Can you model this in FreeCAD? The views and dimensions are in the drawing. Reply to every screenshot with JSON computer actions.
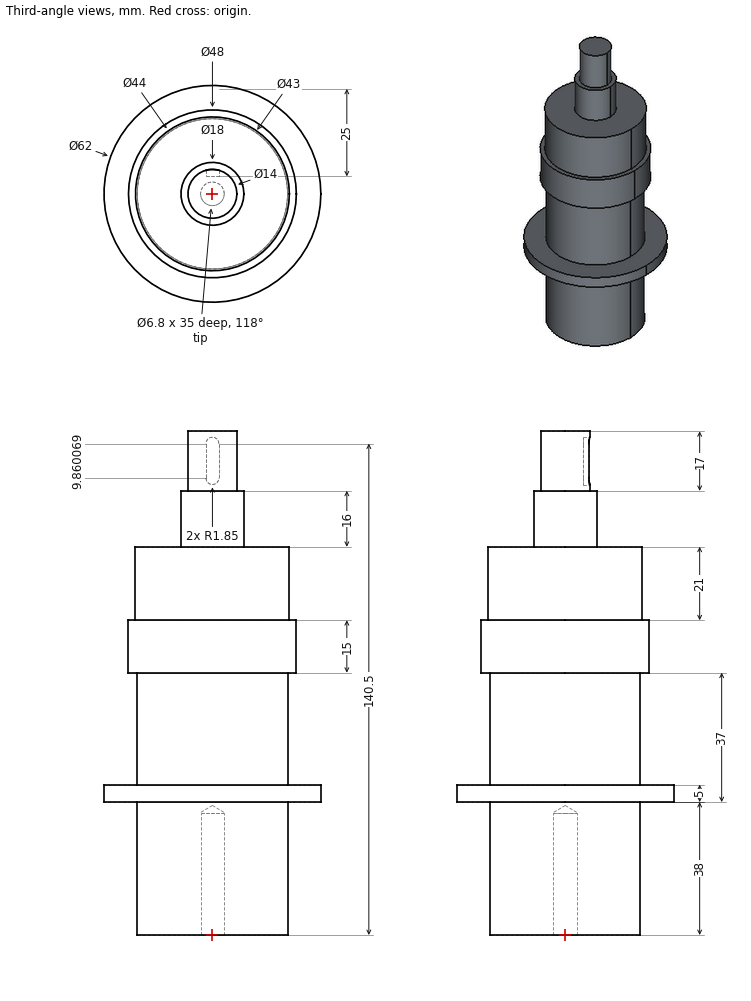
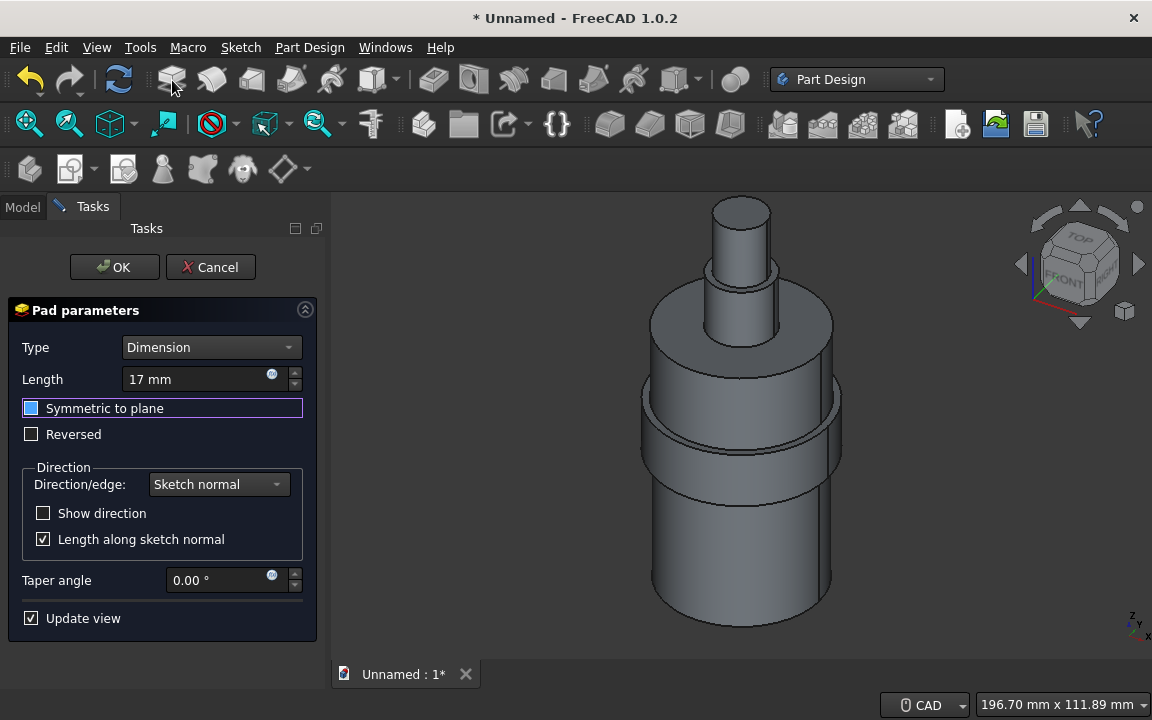
{"action": "left_click", "coordinate": [115, 267]}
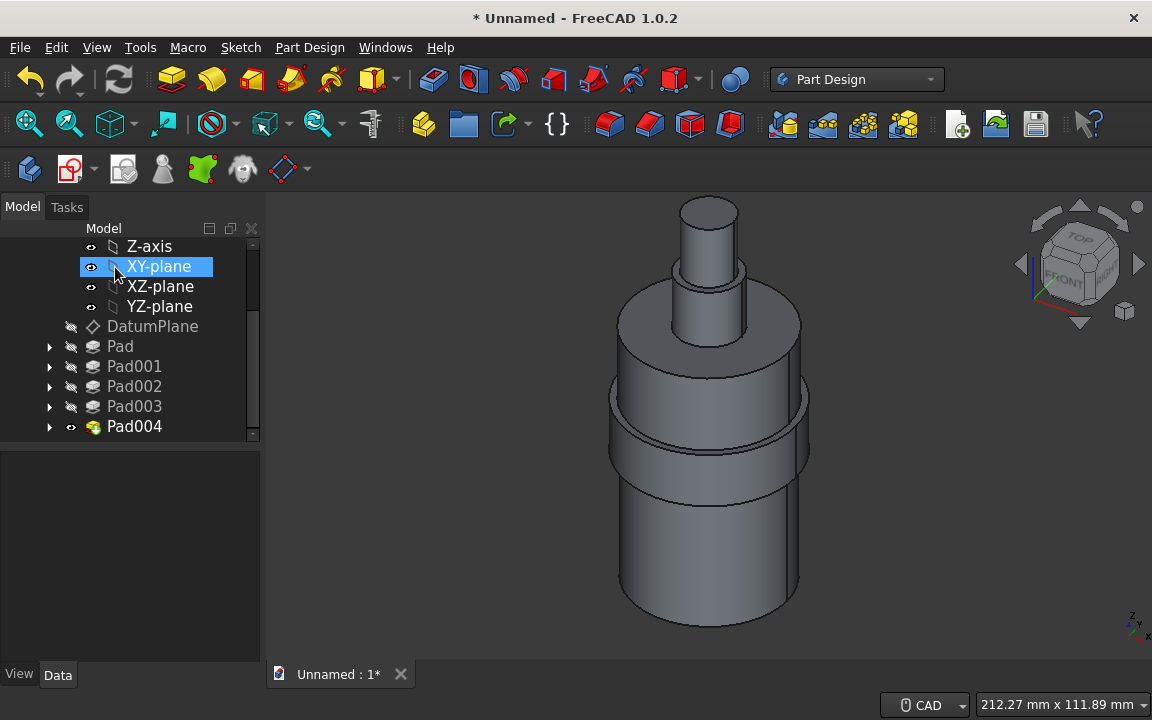
{"action": "left_click", "coordinate": [30, 124]}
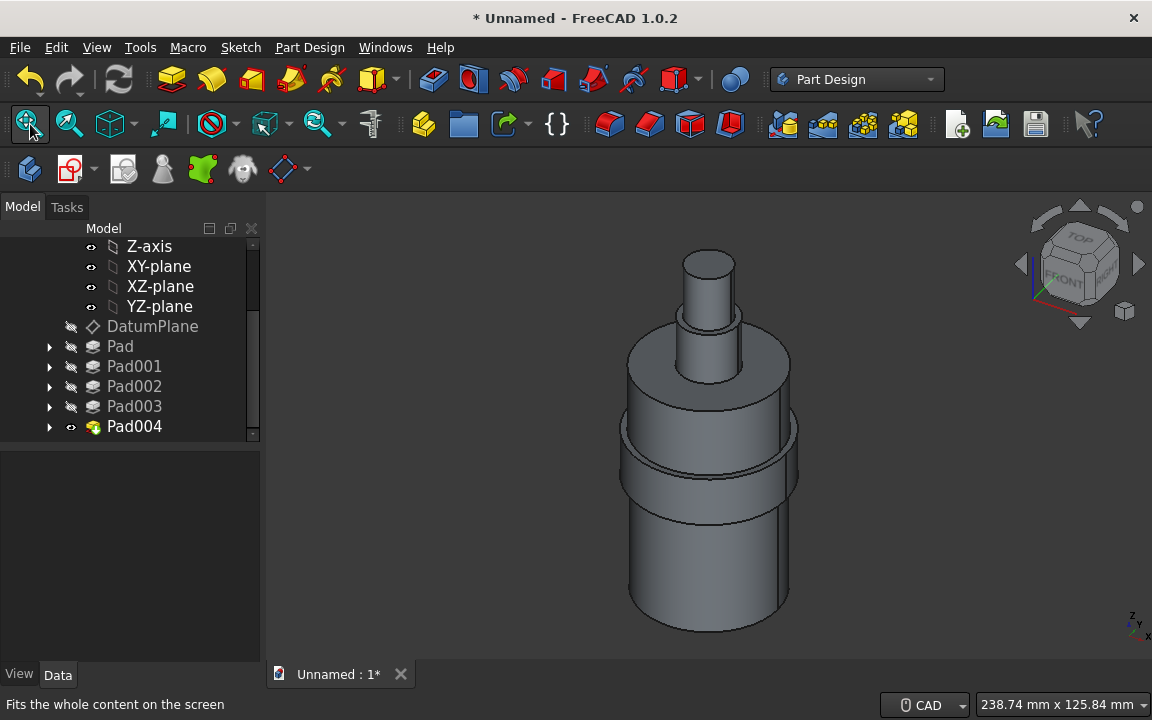
{"action": "scroll", "coordinate": [160, 342], "scroll_direction": "down", "scroll_amount": 3}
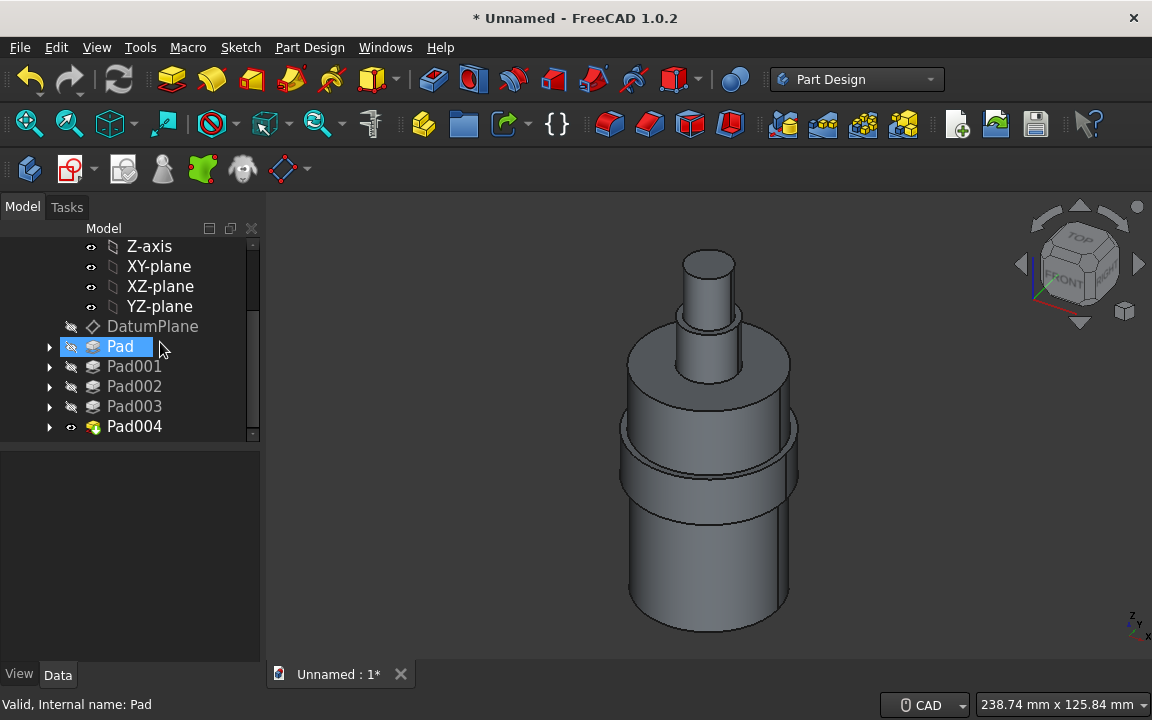
{"action": "scroll", "coordinate": [160, 342], "scroll_direction": "up", "scroll_amount": 15}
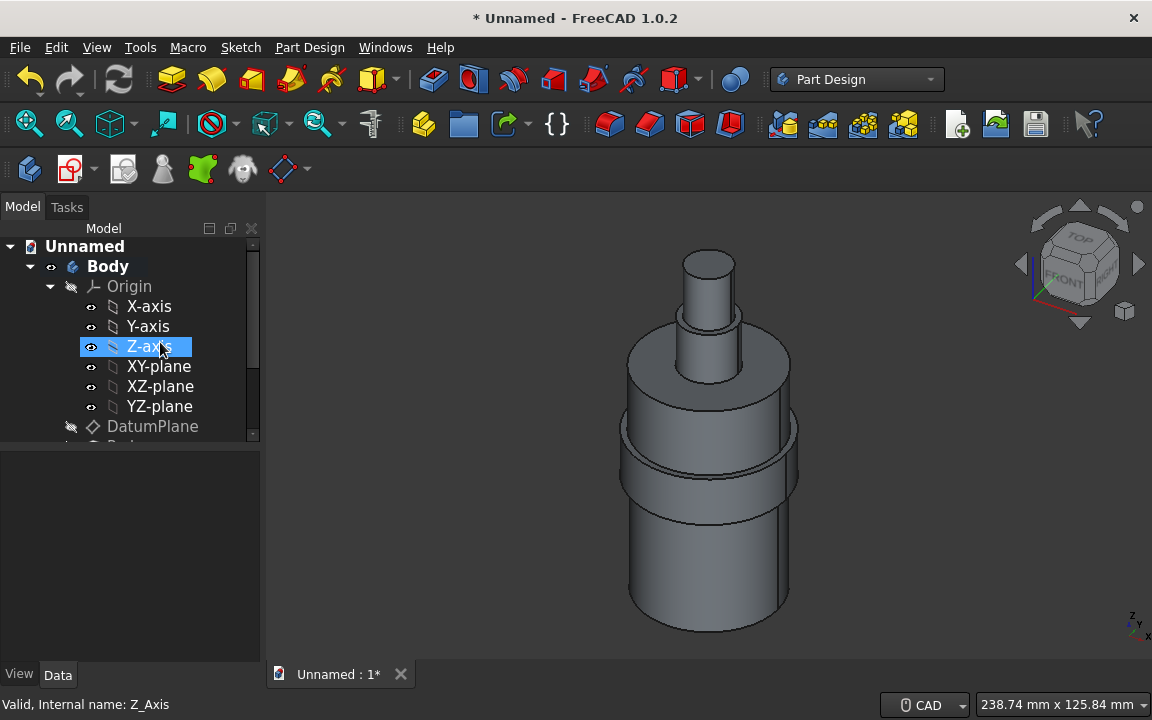
{"action": "left_click", "coordinate": [136, 387]}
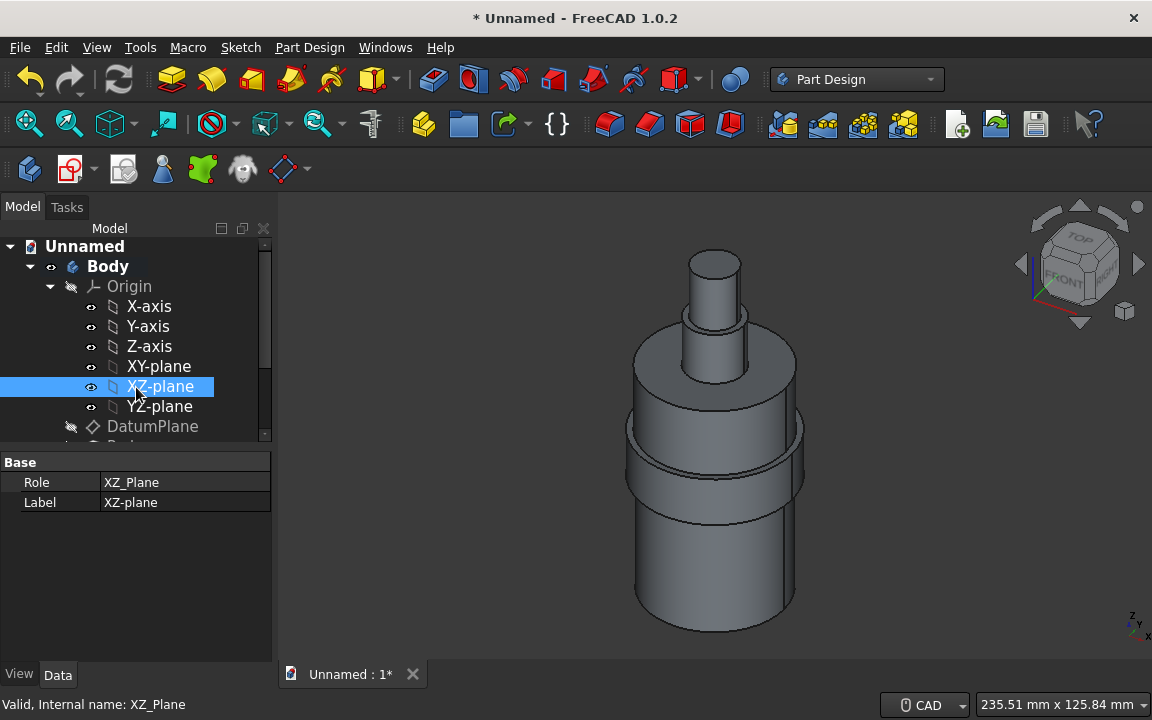
{"action": "left_click", "coordinate": [284, 170]}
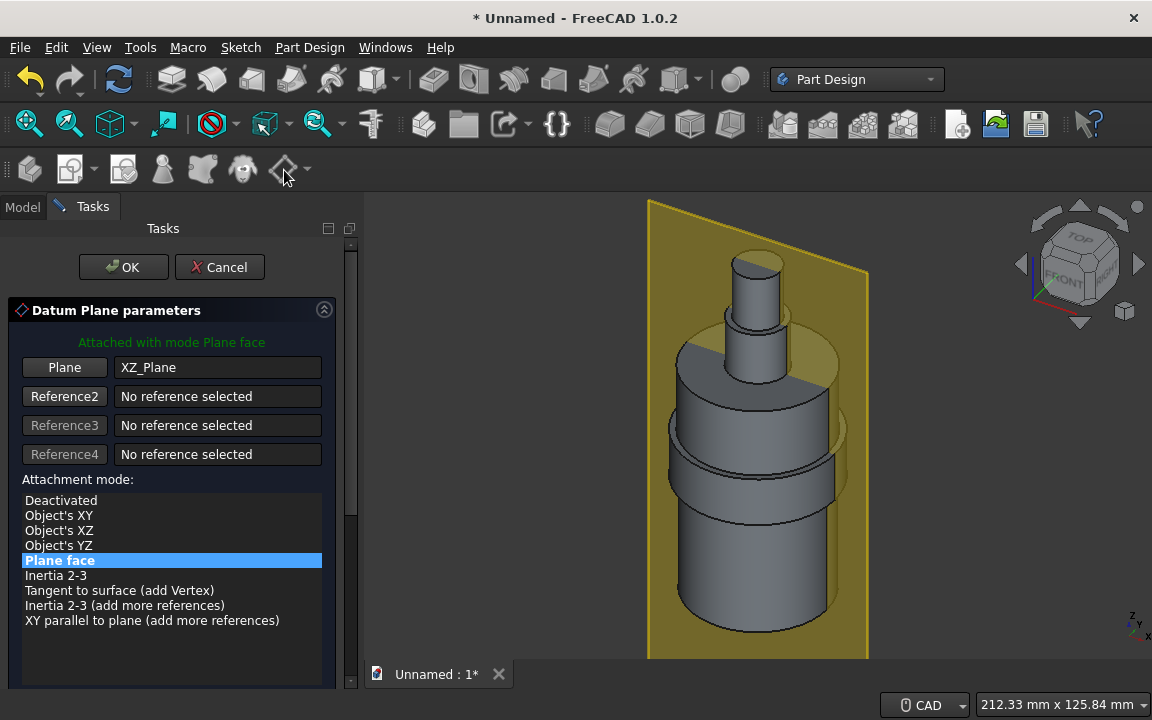
{"action": "scroll", "coordinate": [351, 463], "scroll_direction": "down", "scroll_amount": 3}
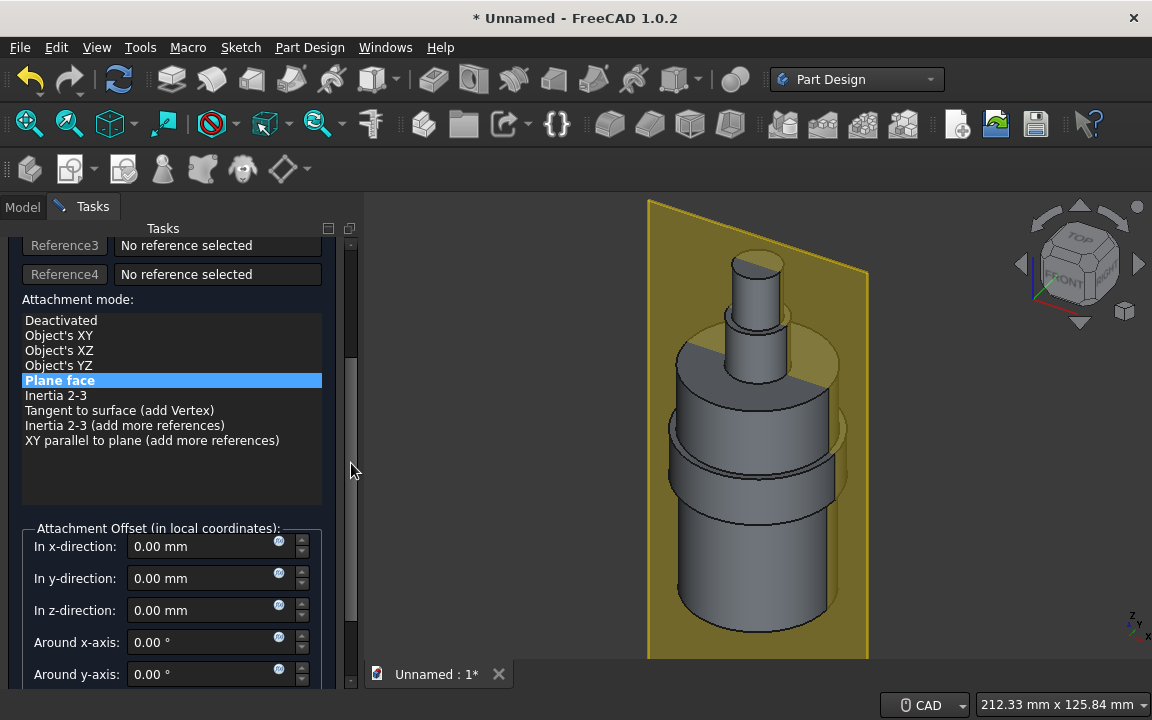
{"action": "triple_click", "coordinate": [210, 610]}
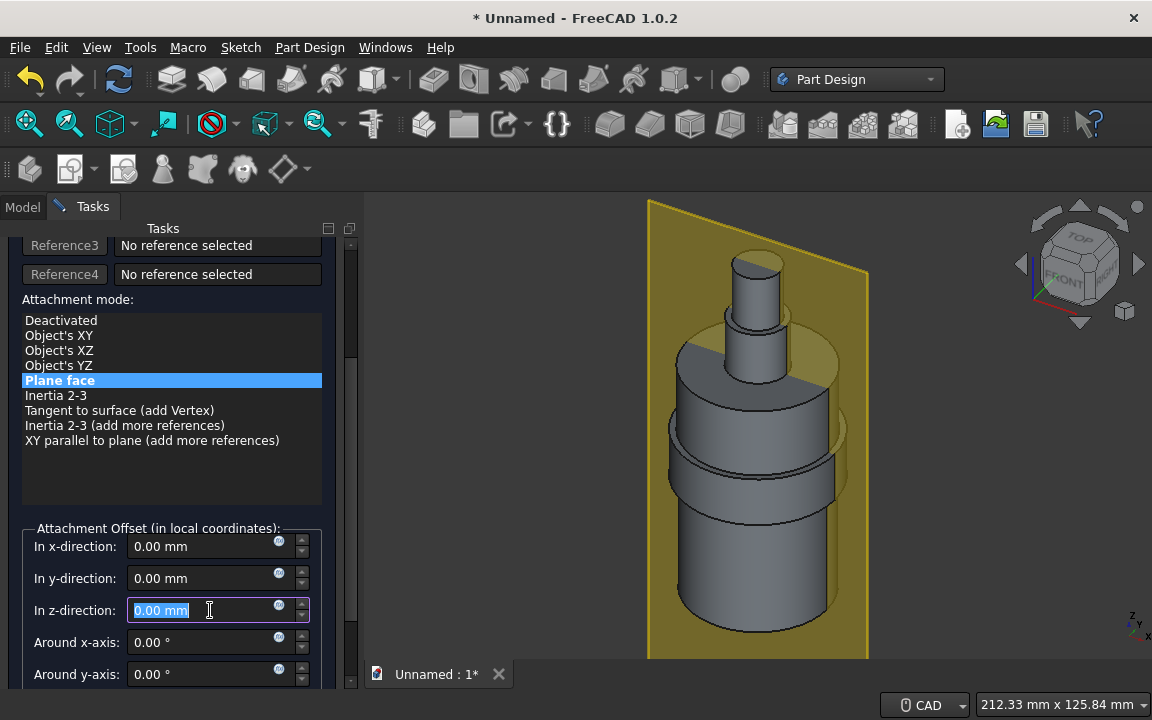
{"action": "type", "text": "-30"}
{"action": "key", "text": "Tab"}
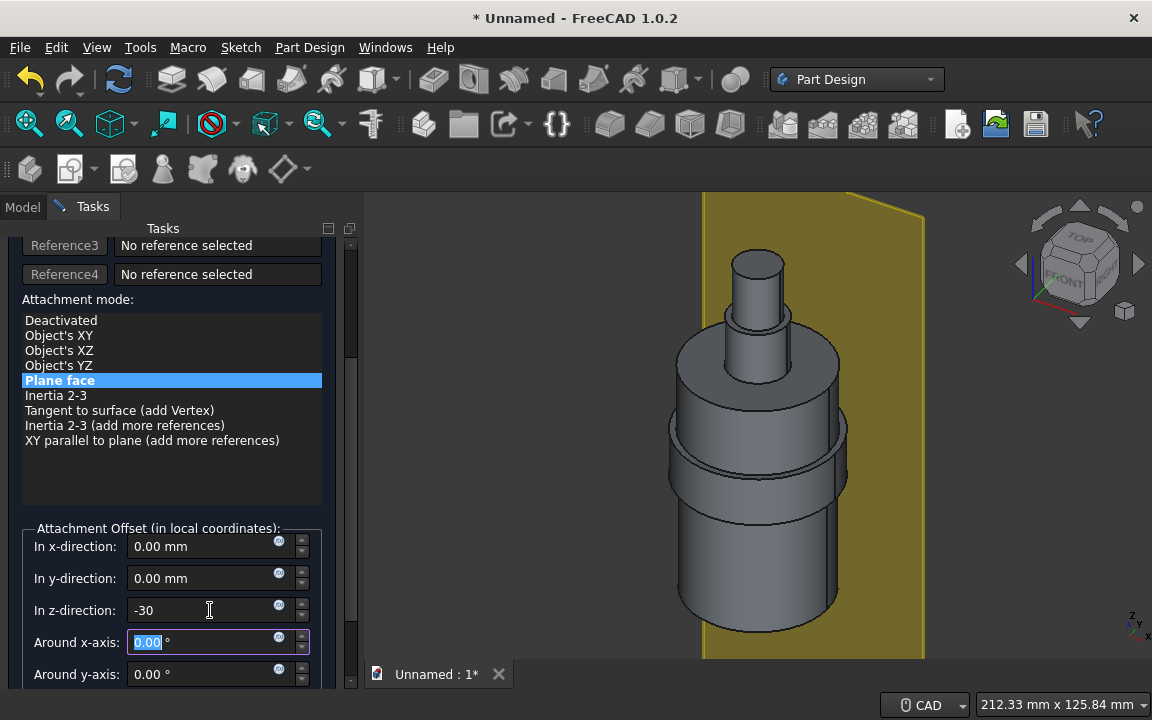
{"action": "scroll", "coordinate": [351, 463], "scroll_direction": "up", "scroll_amount": 4}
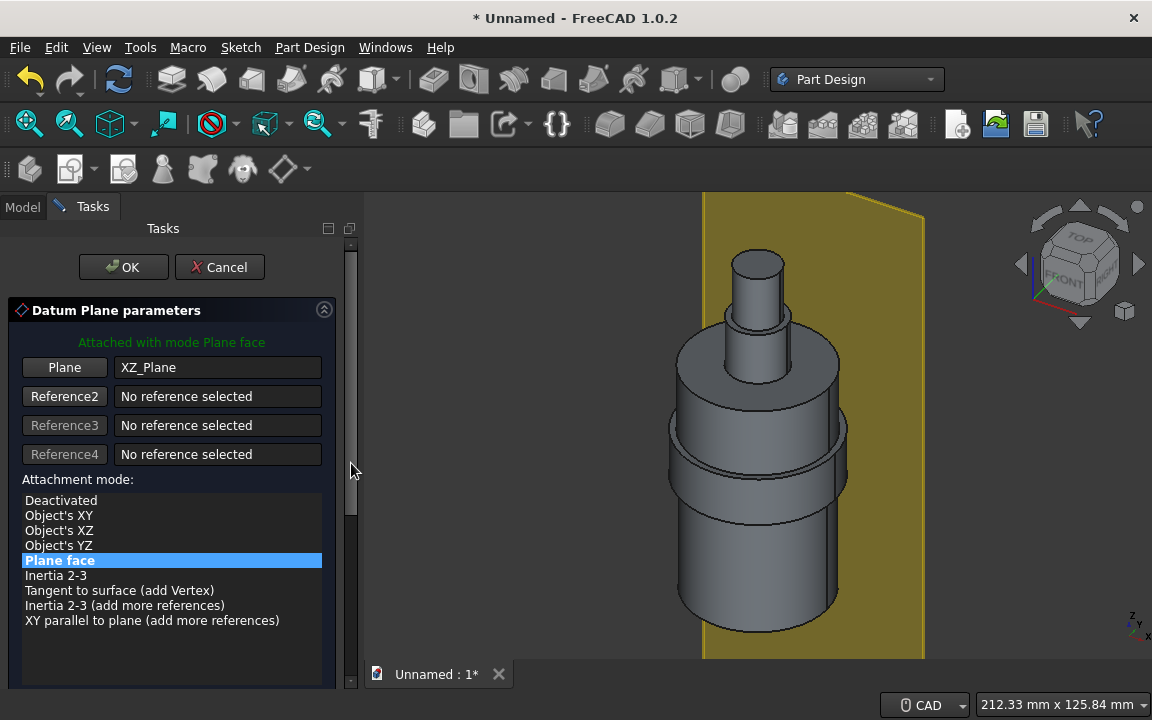
{"action": "left_click", "coordinate": [124, 267]}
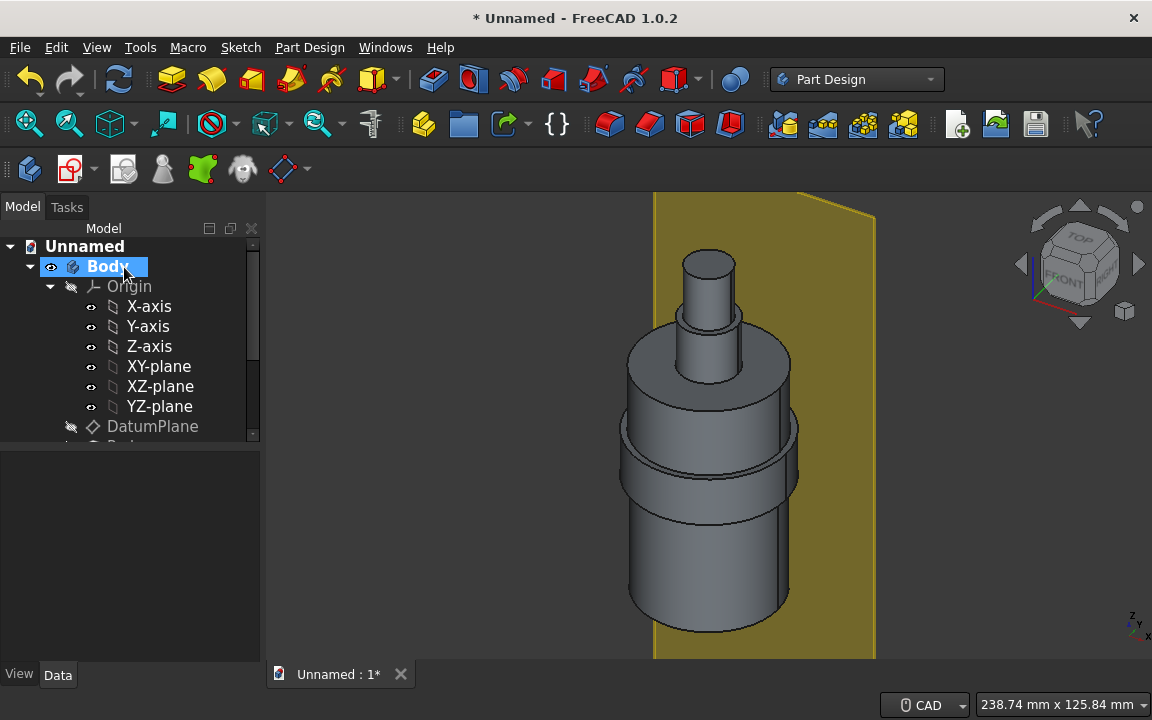
{"action": "scroll", "coordinate": [100, 342], "scroll_direction": "down", "scroll_amount": 3}